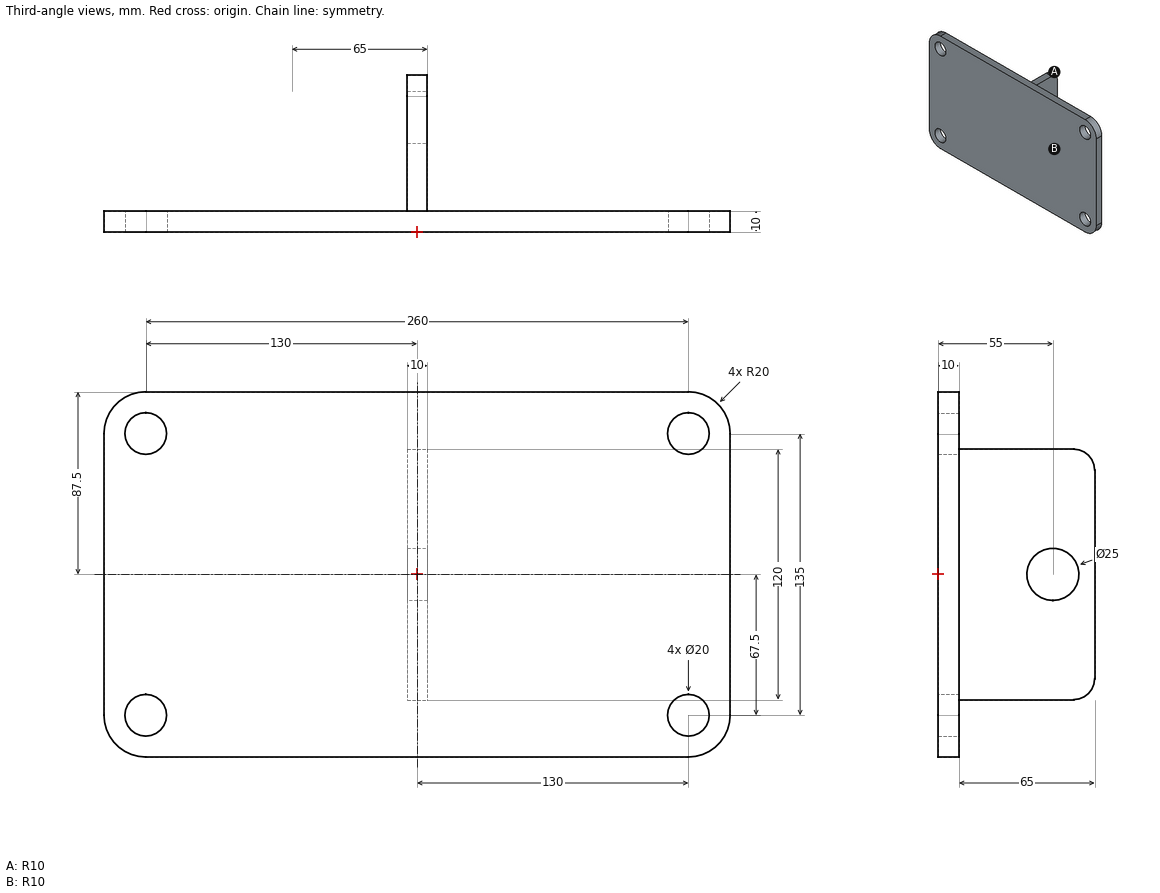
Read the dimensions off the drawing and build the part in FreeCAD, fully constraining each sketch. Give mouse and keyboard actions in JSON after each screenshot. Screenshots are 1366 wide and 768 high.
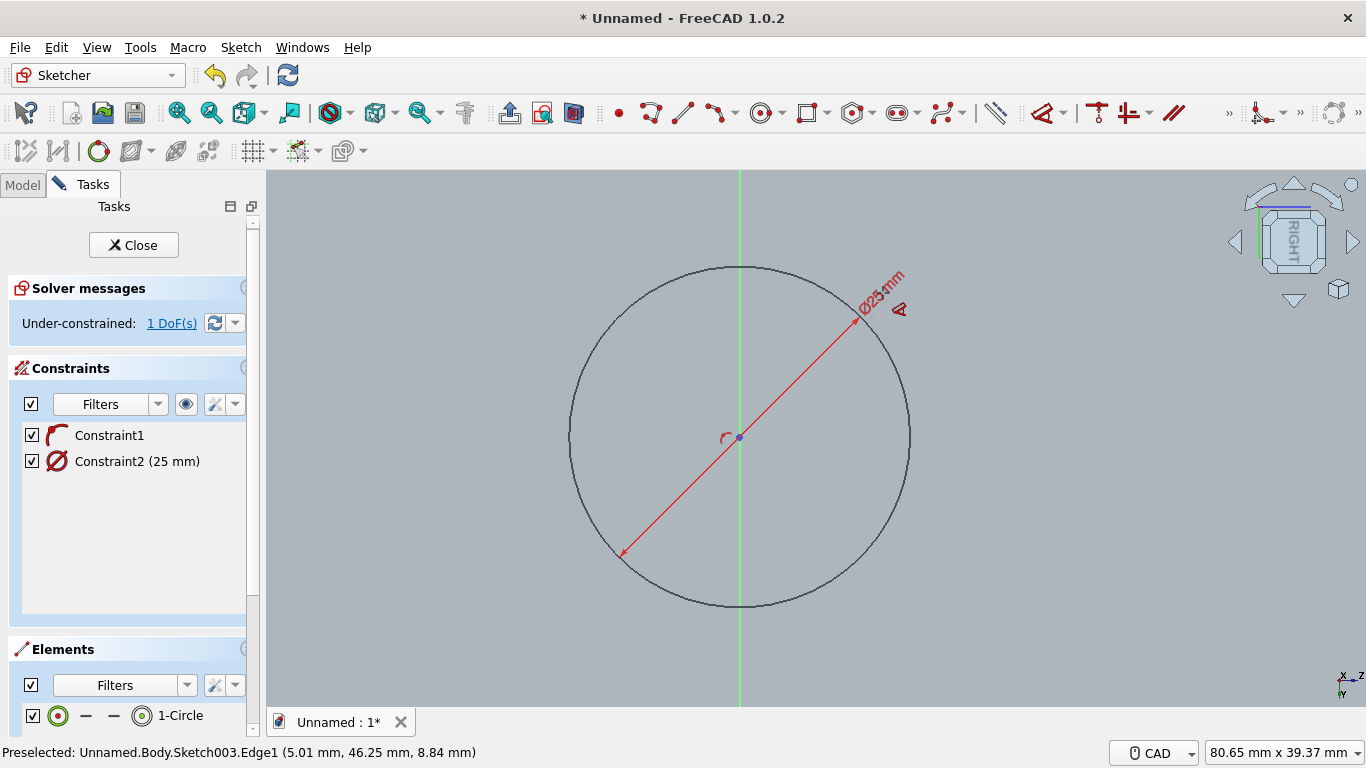
{"action": "left_click", "coordinate": [740, 437]}
{"action": "left_click", "coordinate": [774, 317]}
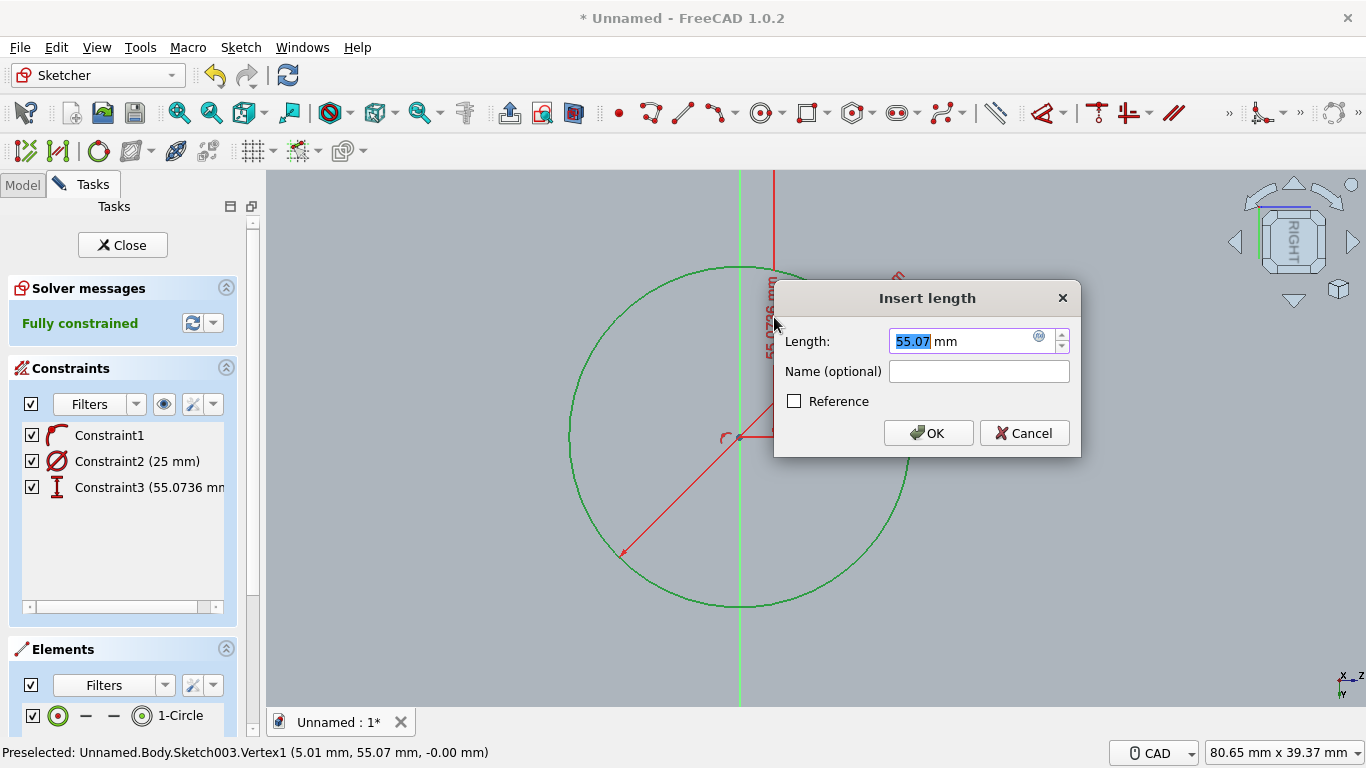
{"action": "type", "text": "55"}
{"action": "key", "text": "Return"}
{"action": "key", "text": "Escape"}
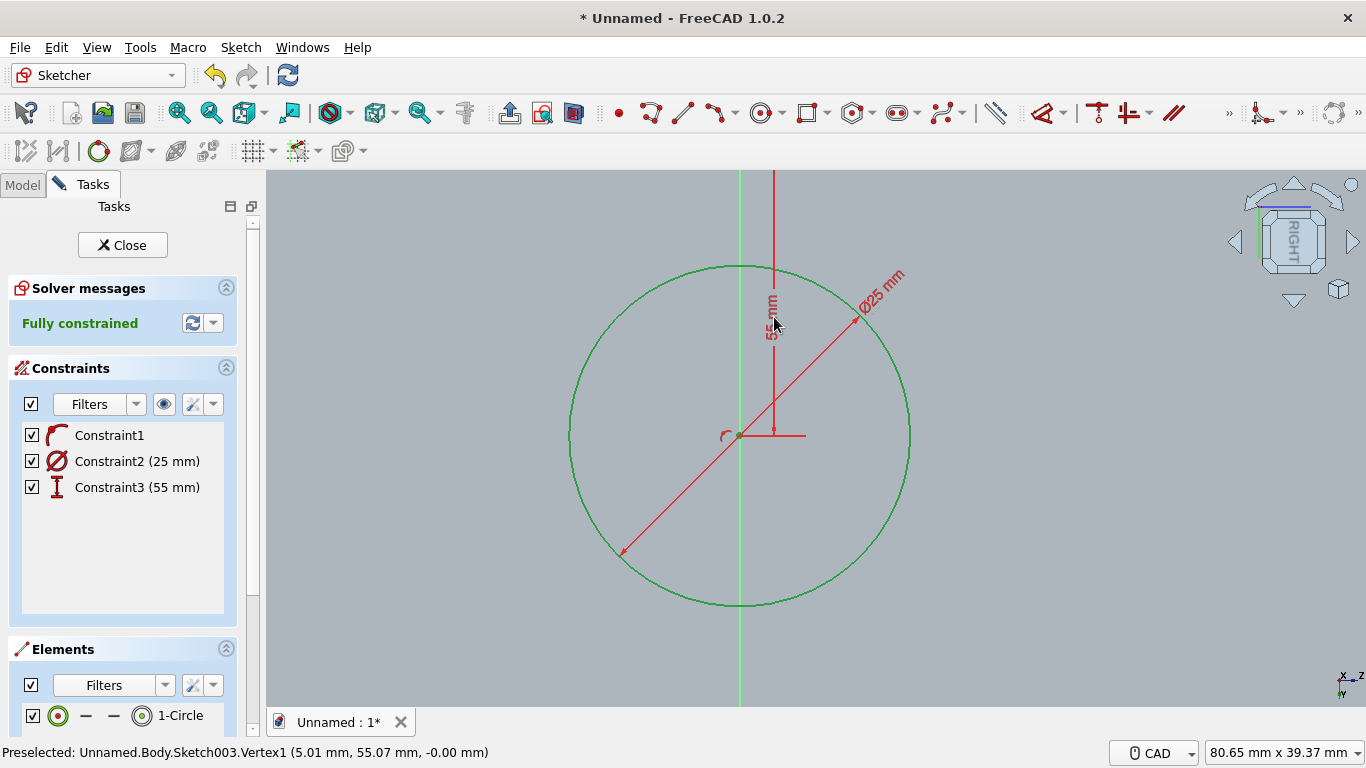
{"action": "left_click", "coordinate": [123, 245]}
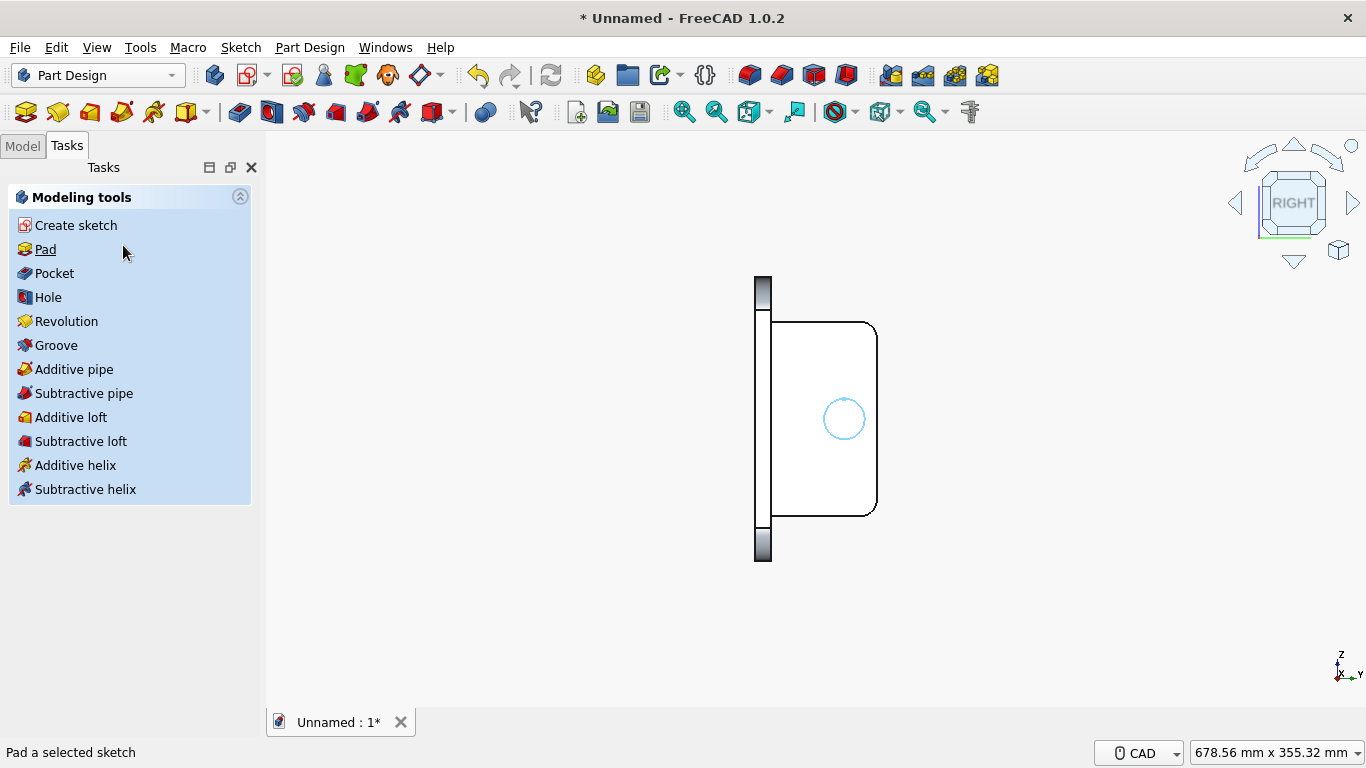
{"action": "left_click", "coordinate": [240, 112]}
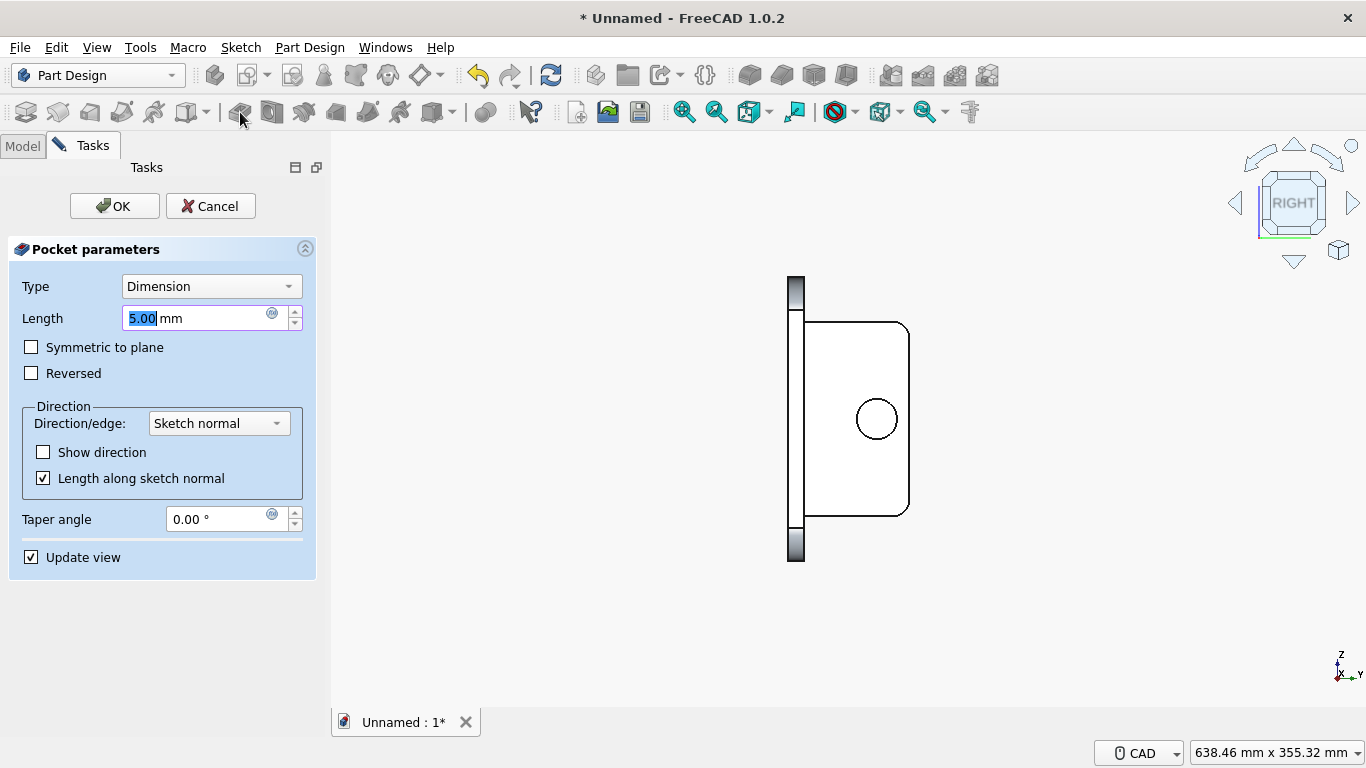
{"action": "type", "text": "65"}
{"action": "key", "text": "Tab"}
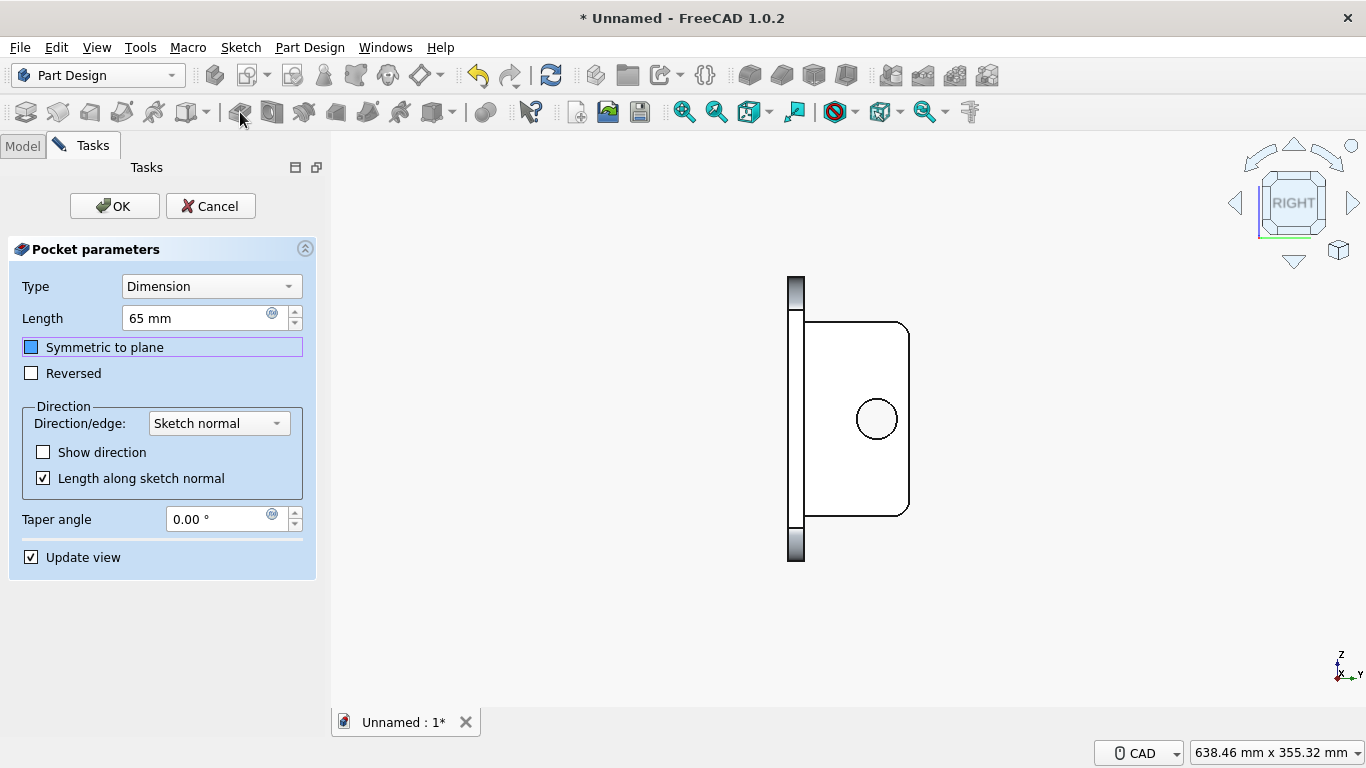
{"action": "left_click", "coordinate": [115, 206]}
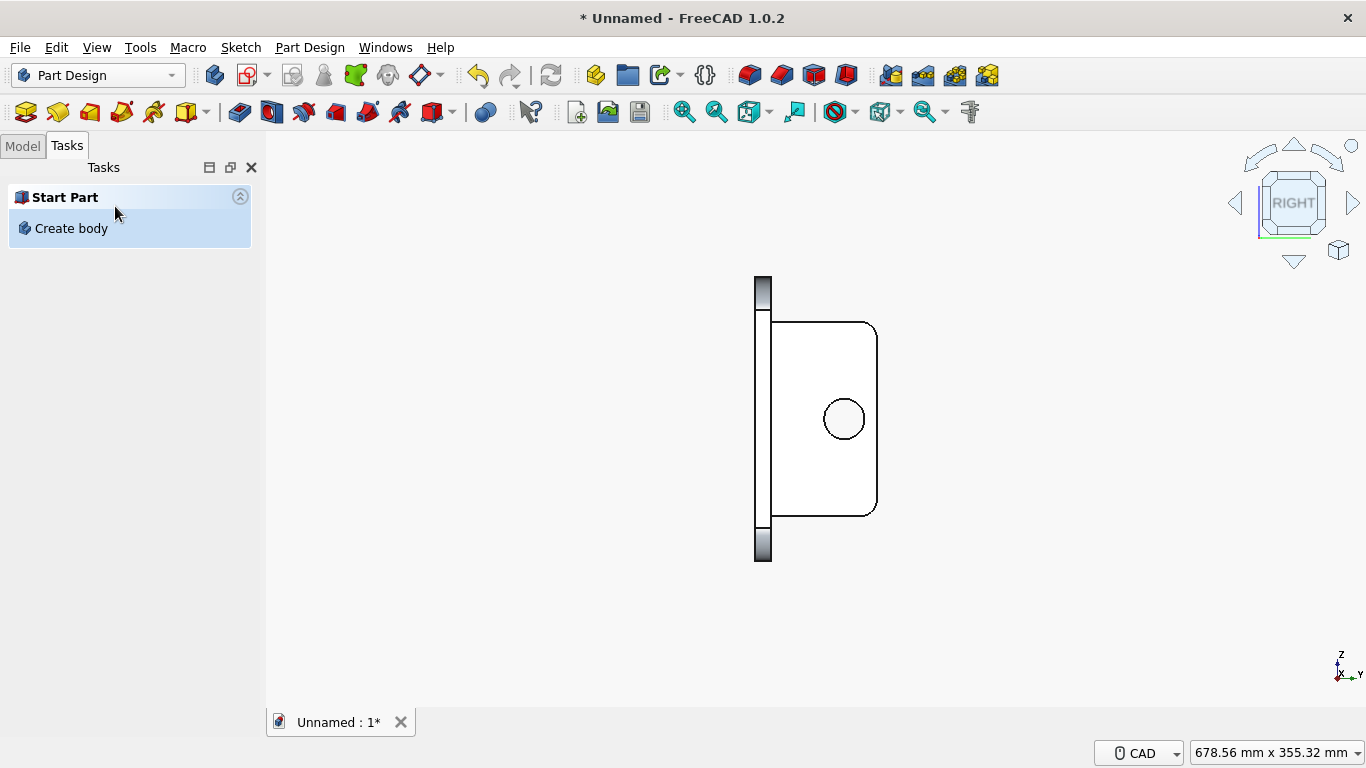
{"action": "key", "text": "0"}